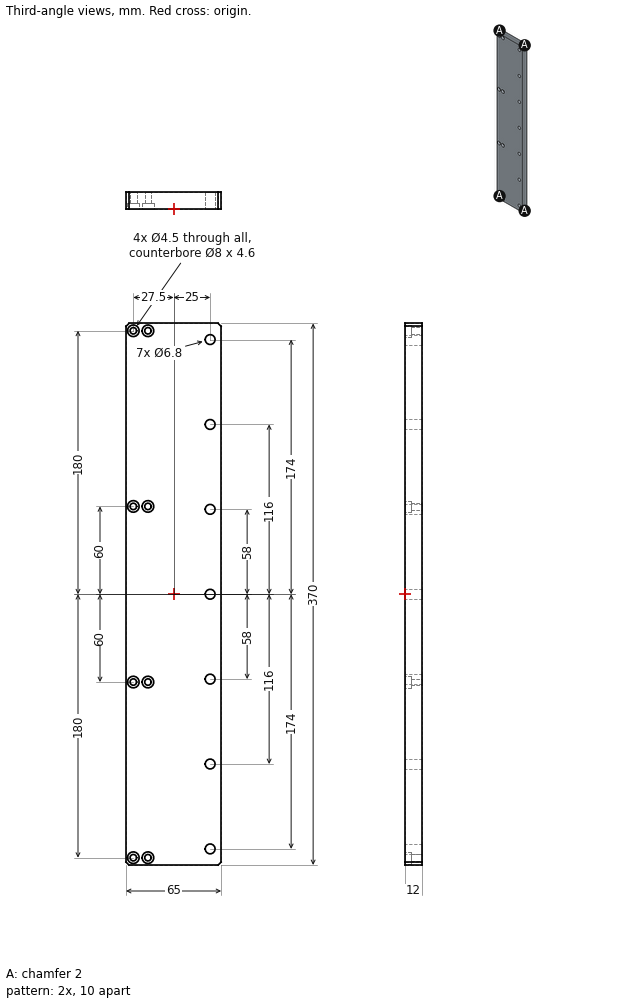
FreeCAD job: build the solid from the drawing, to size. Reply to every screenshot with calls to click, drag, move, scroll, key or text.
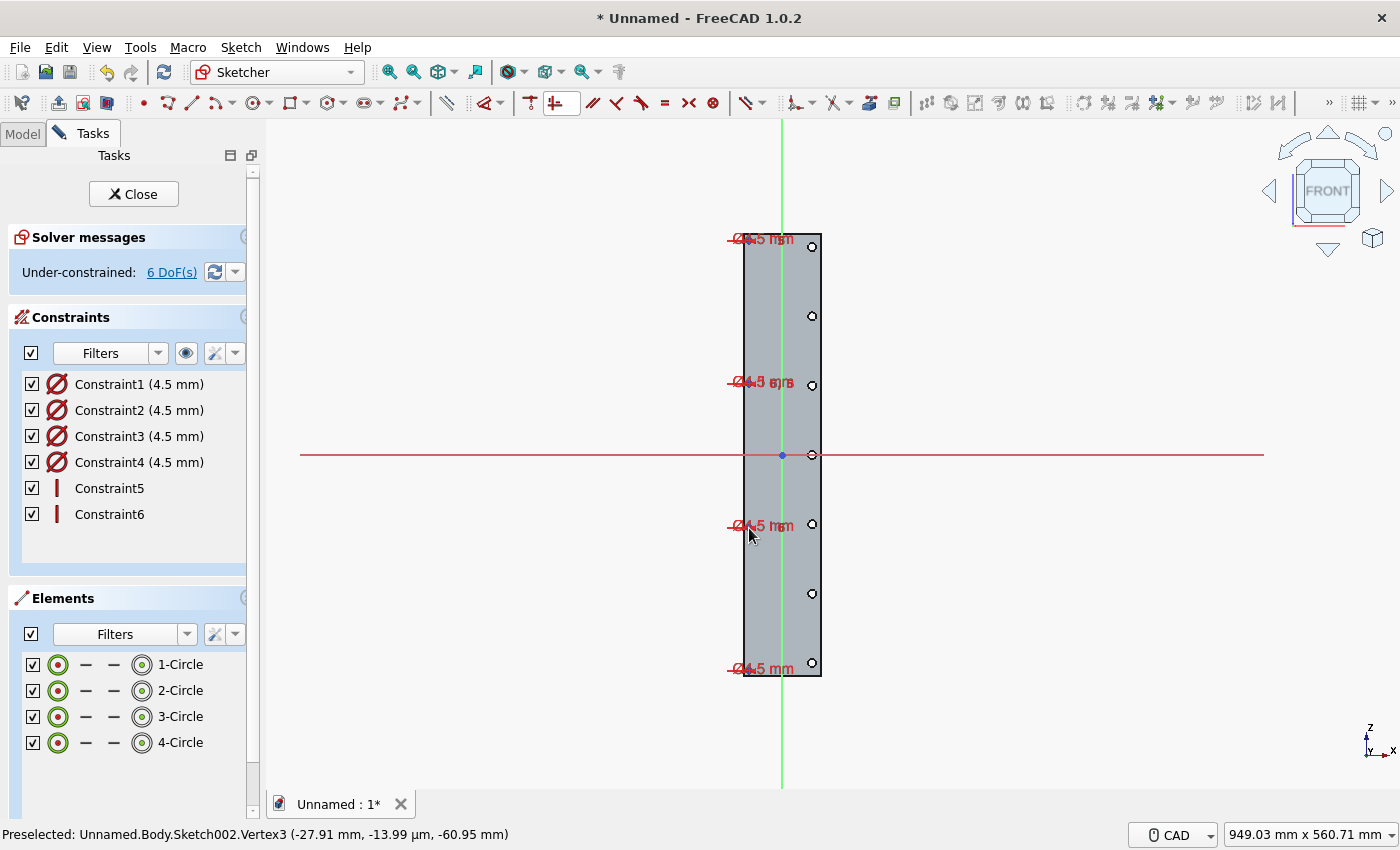
click(749, 528)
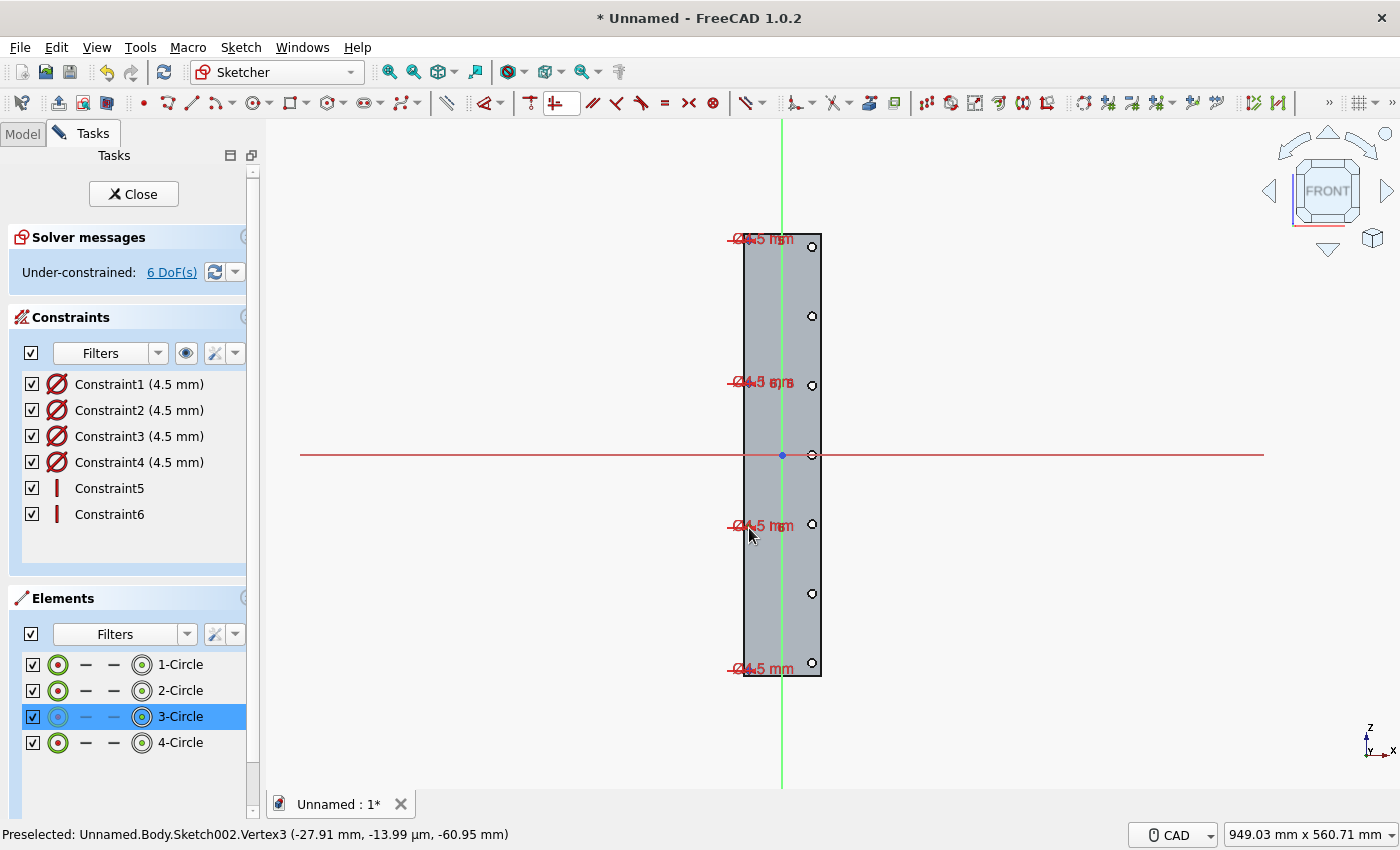
click(749, 671)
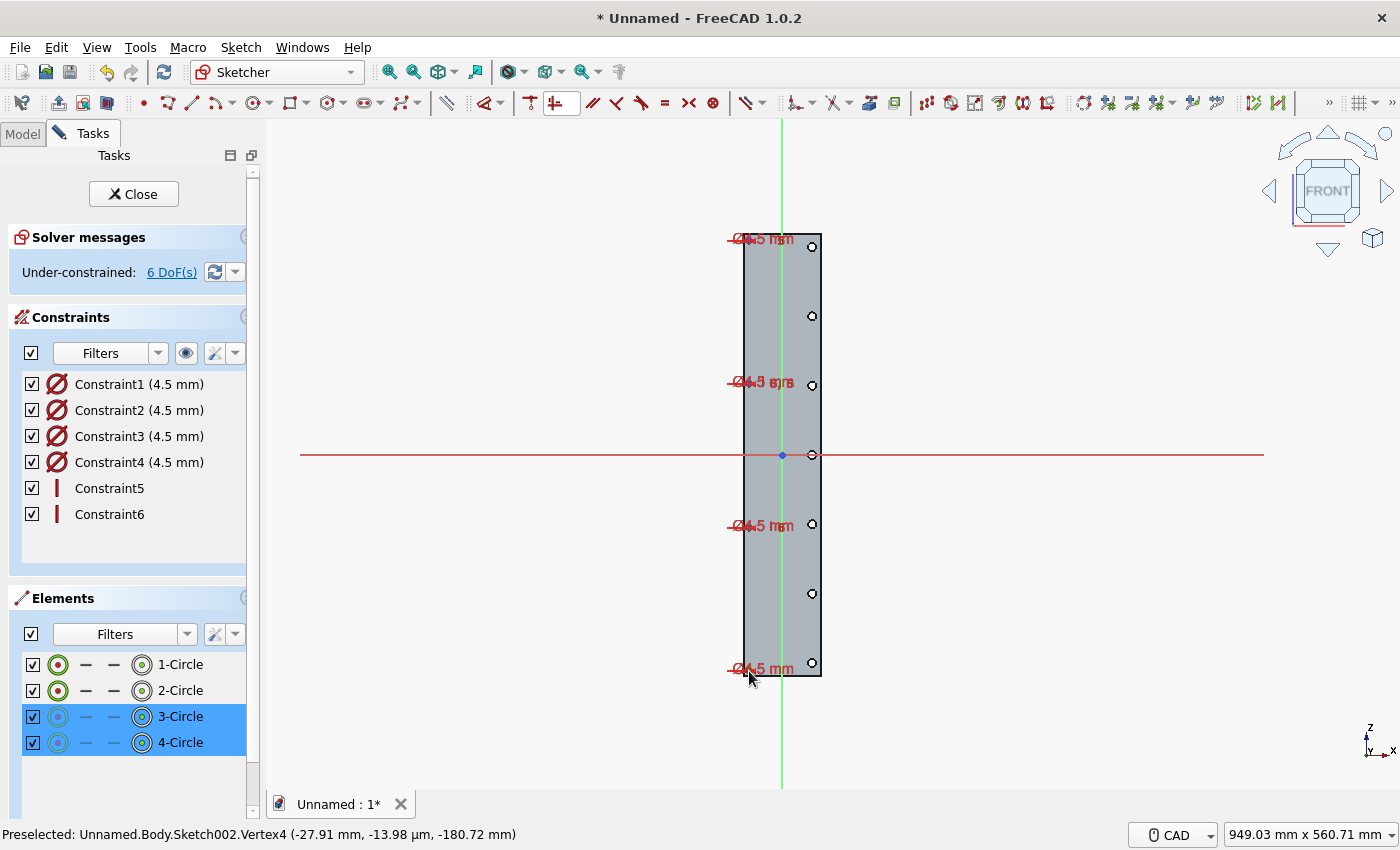
key(v)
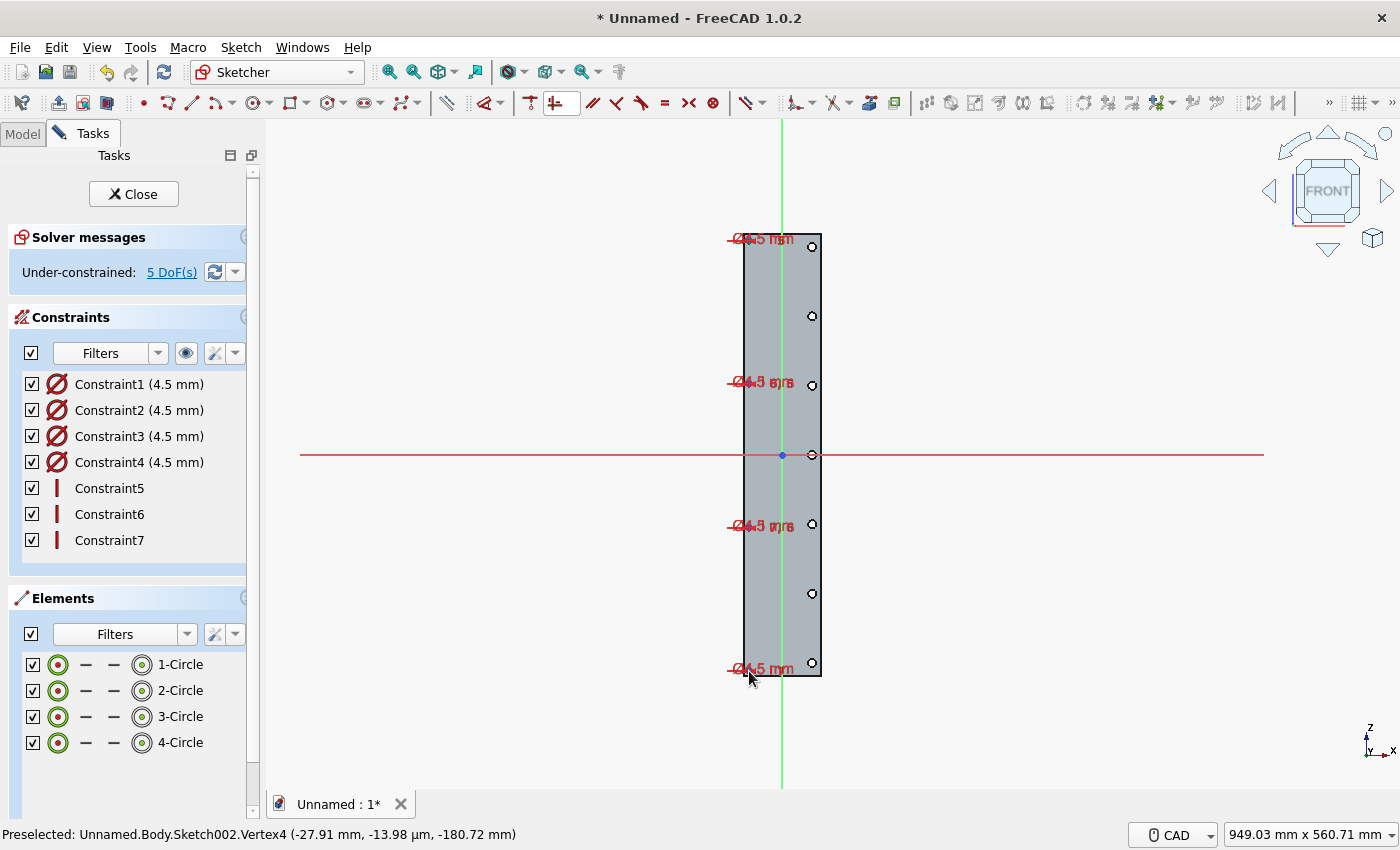
key(d)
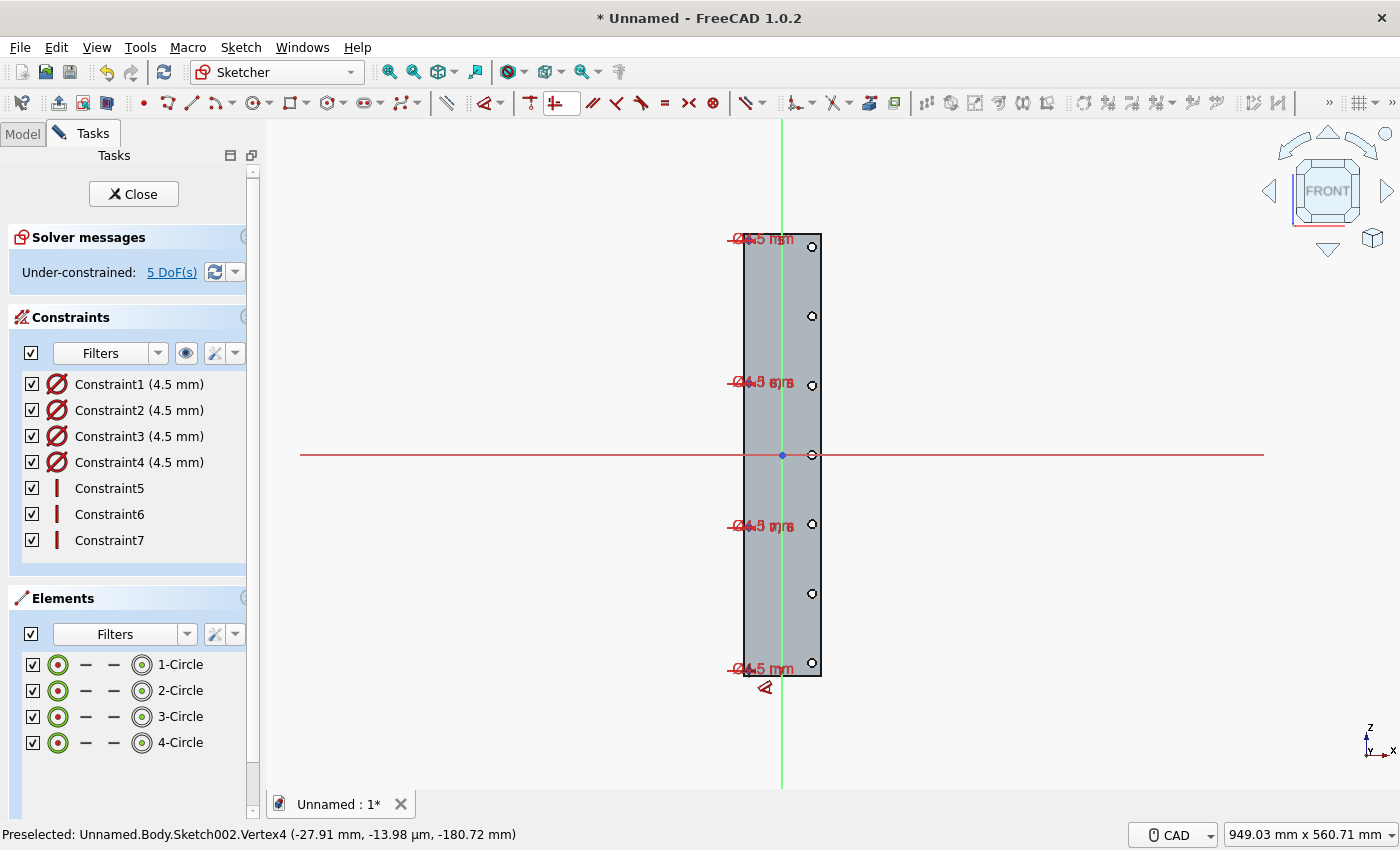
click(749, 384)
click(816, 419)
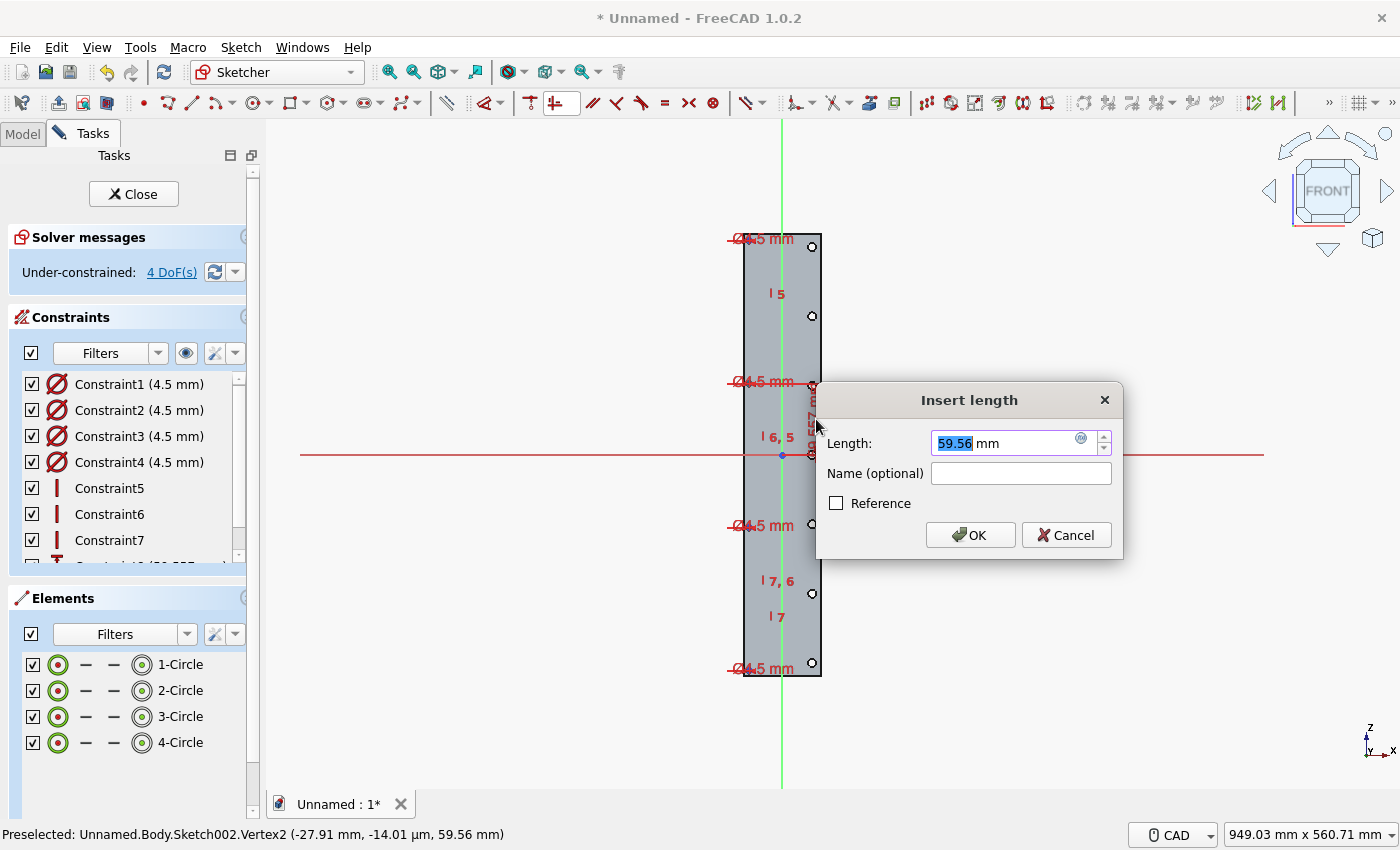
text(60)
key(Return)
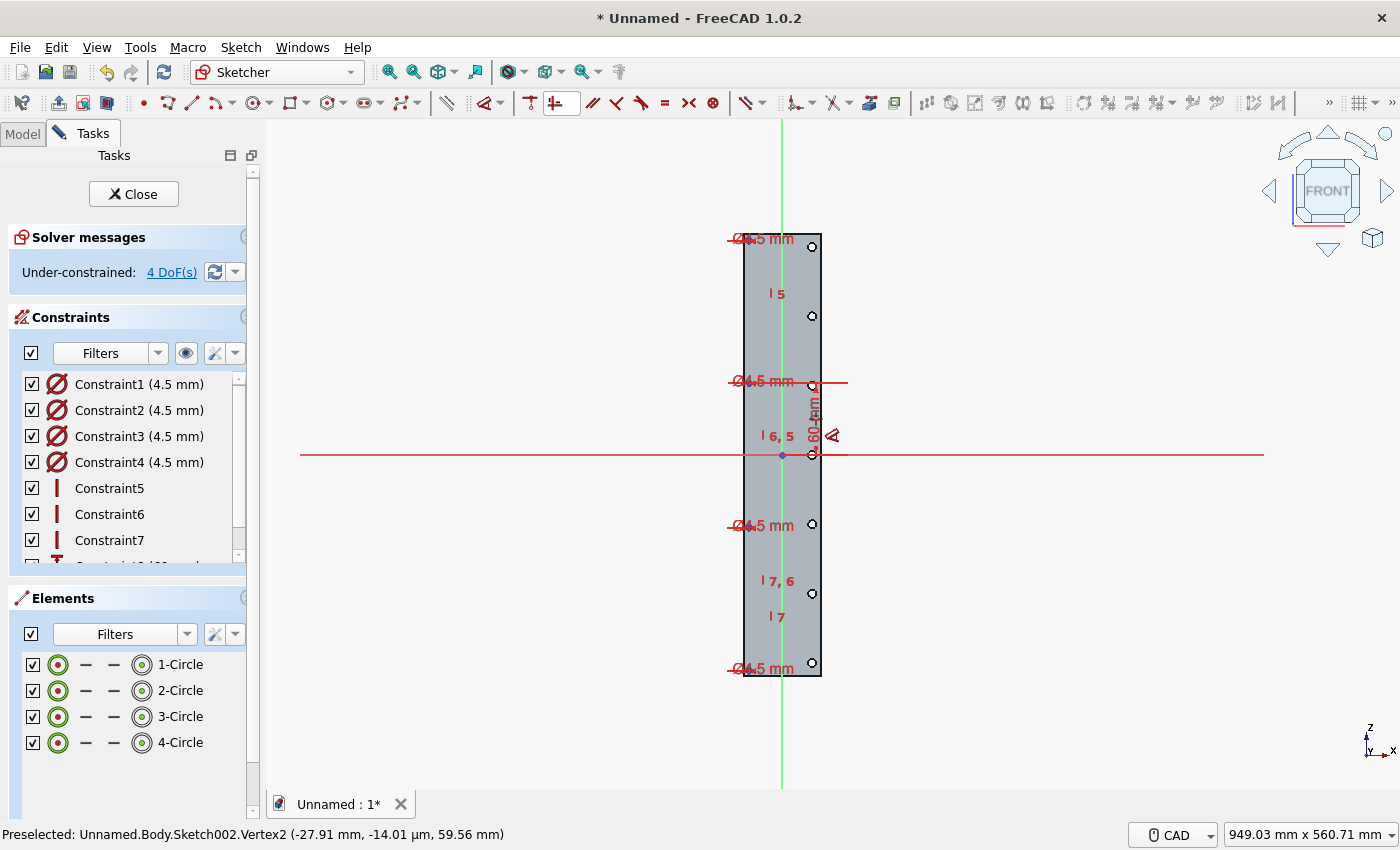
click(749, 528)
click(816, 491)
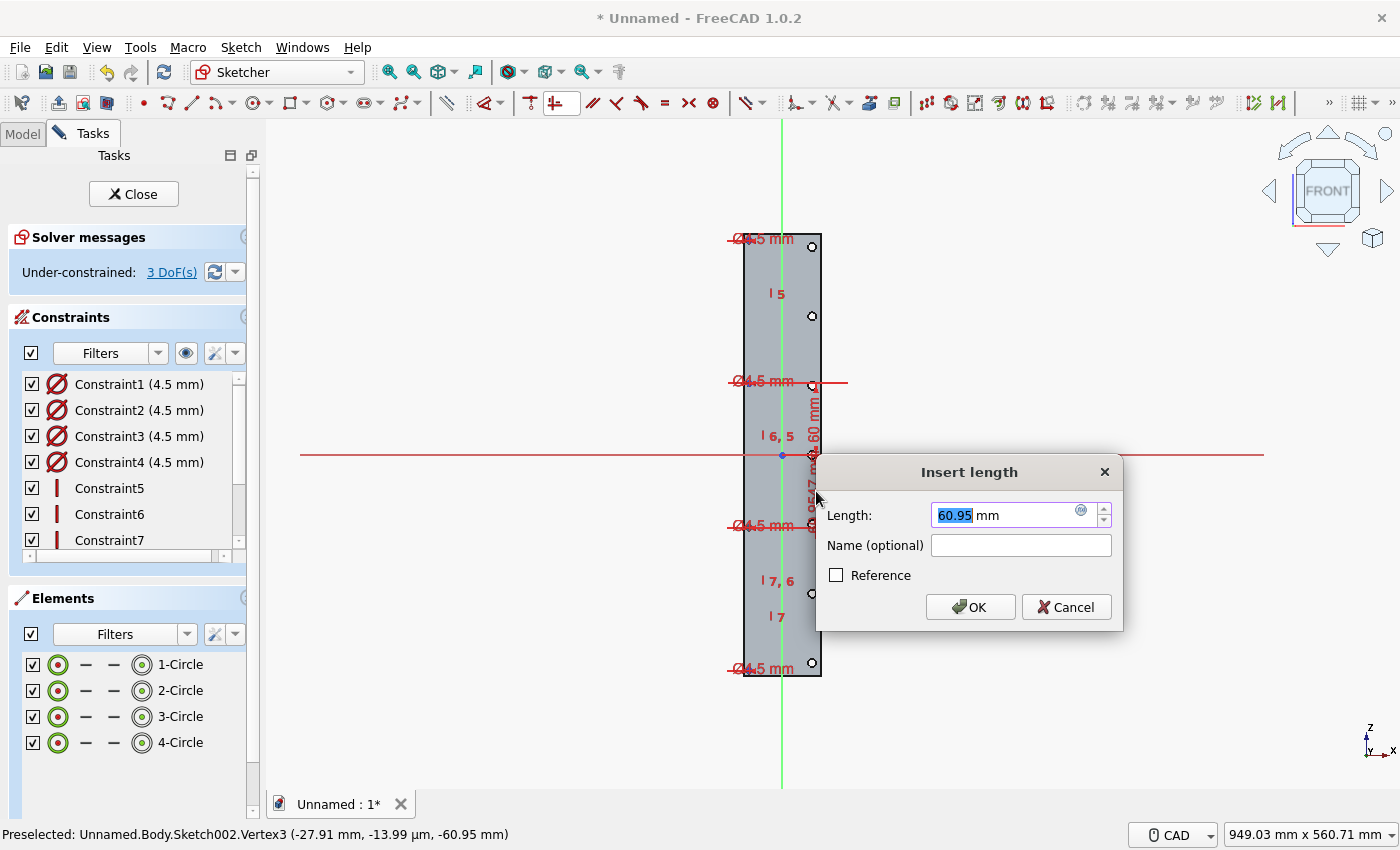
text(60)
key(Return)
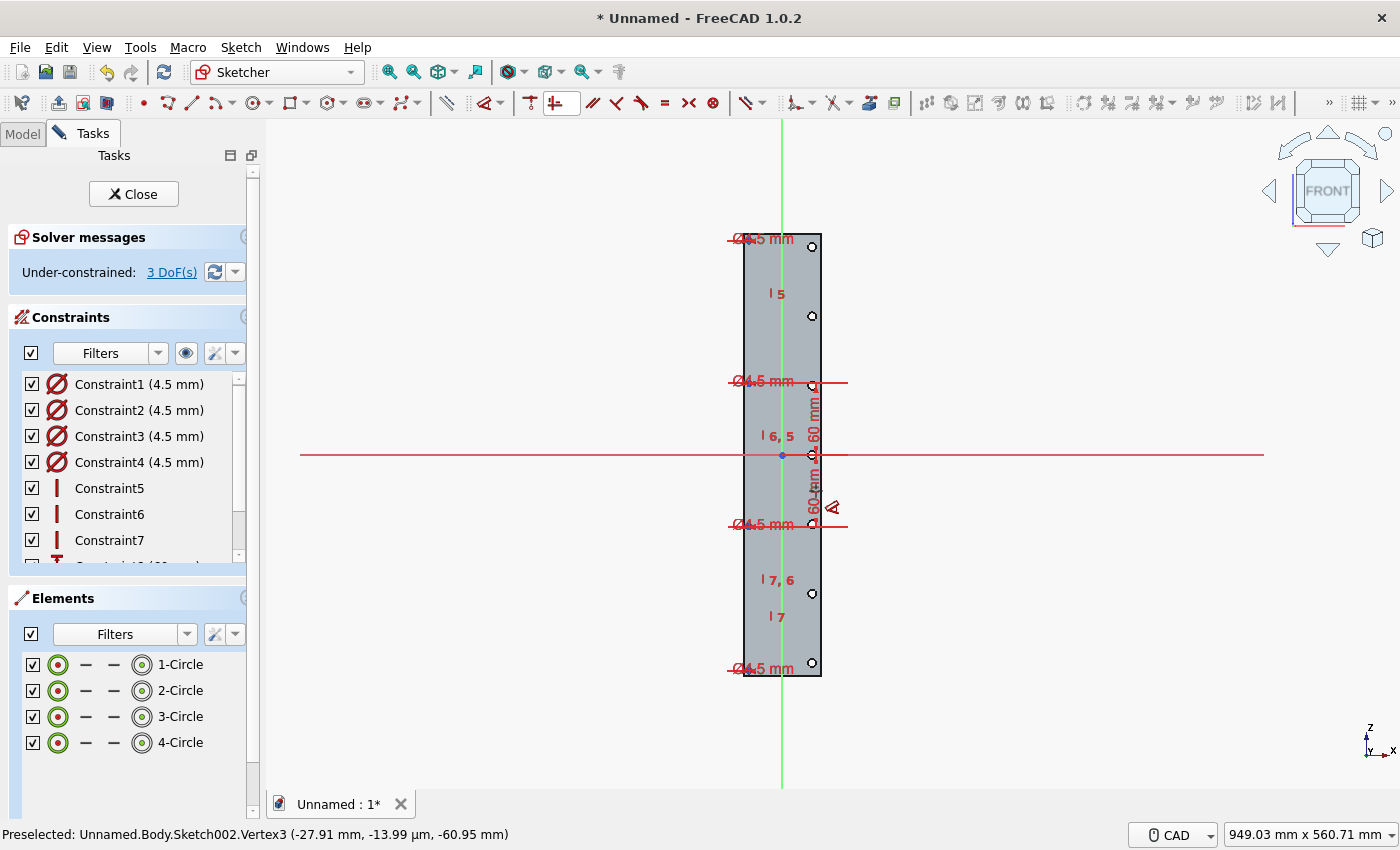
click(749, 241)
click(816, 348)